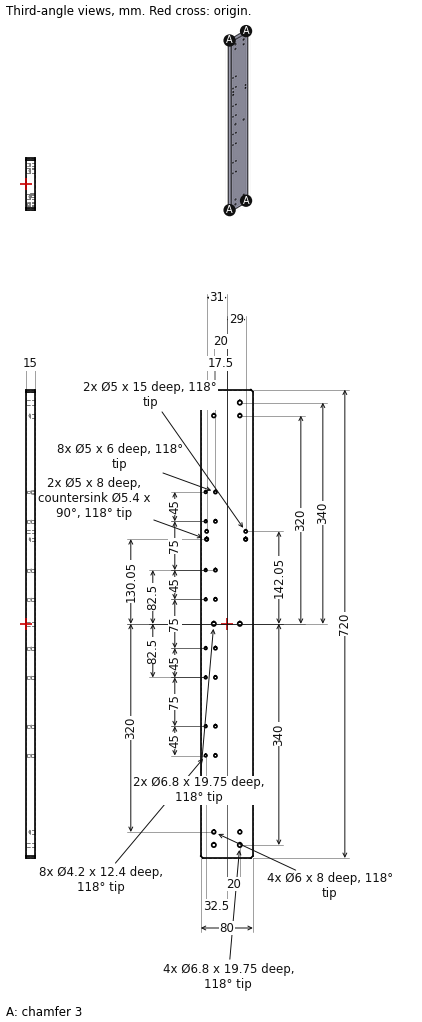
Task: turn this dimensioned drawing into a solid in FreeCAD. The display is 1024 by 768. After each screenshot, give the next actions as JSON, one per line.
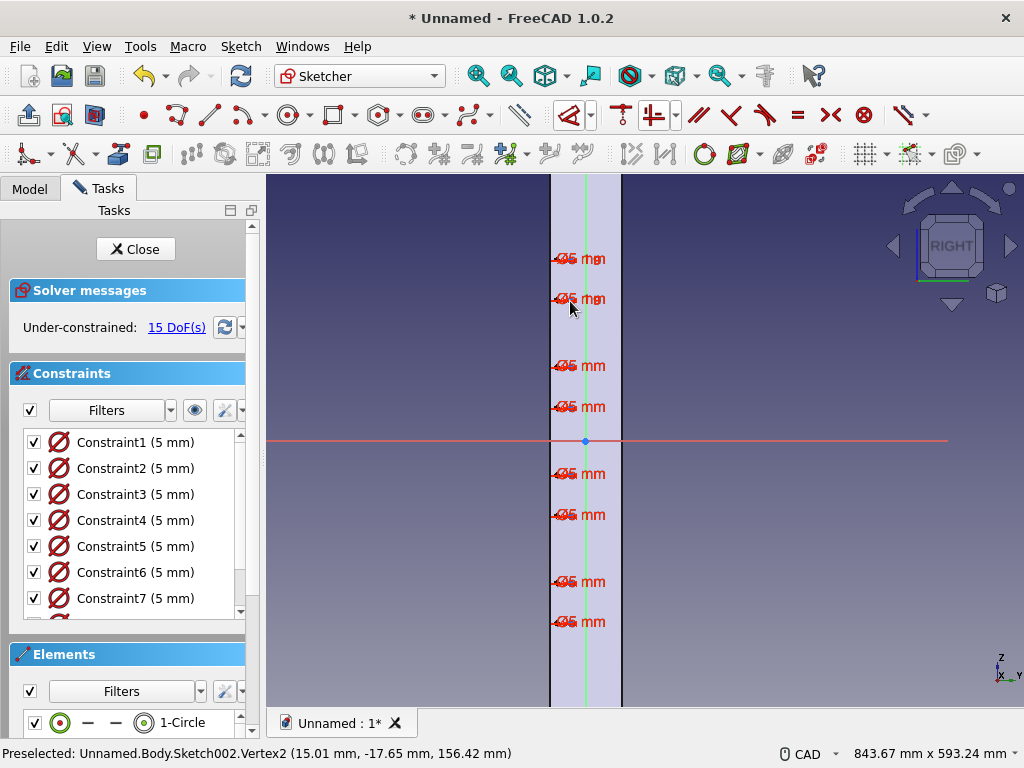
{"action": "left_click", "coordinate": [570, 301]}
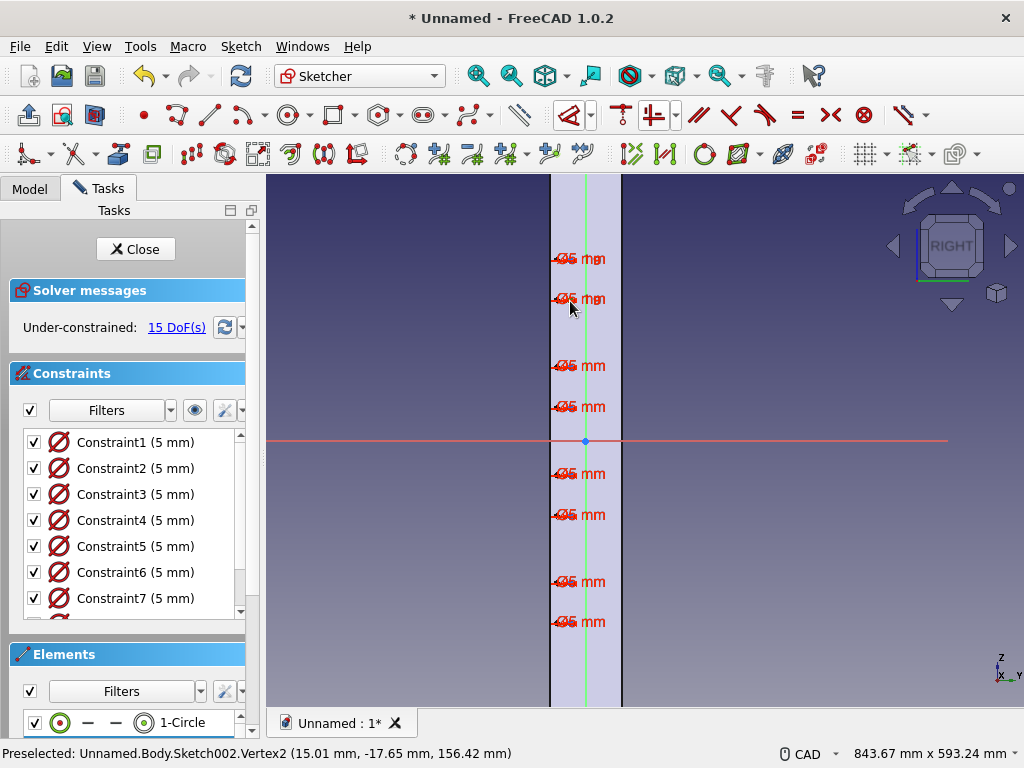
{"action": "left_click", "coordinate": [570, 368]}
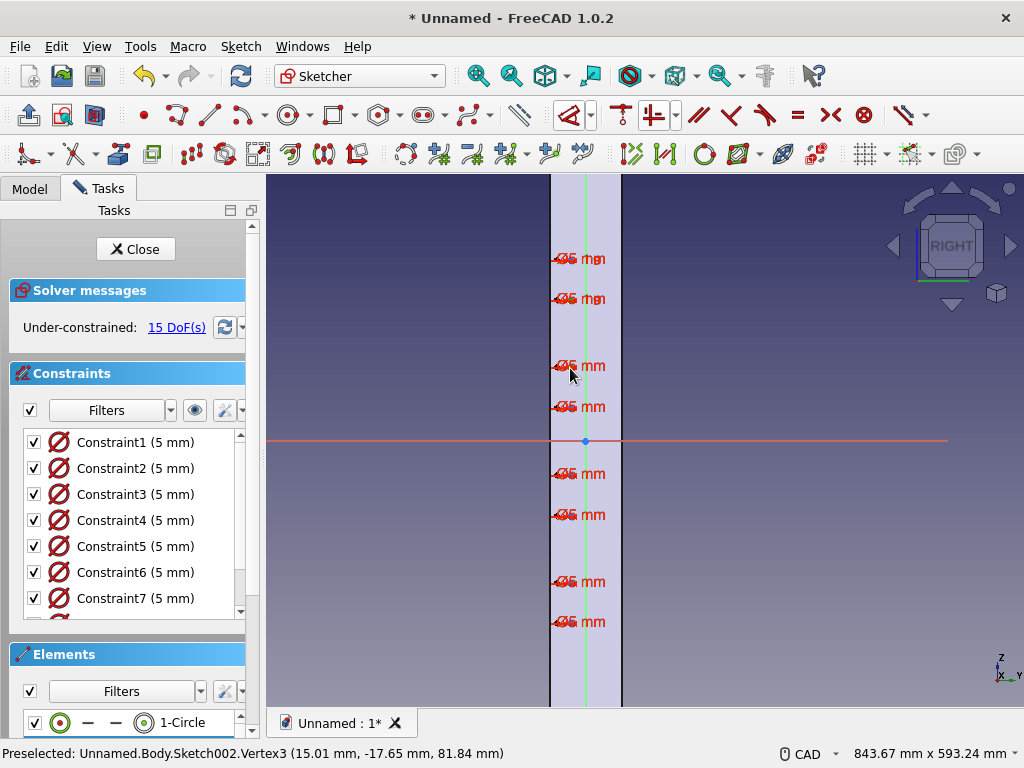
{"action": "key", "text": "v"}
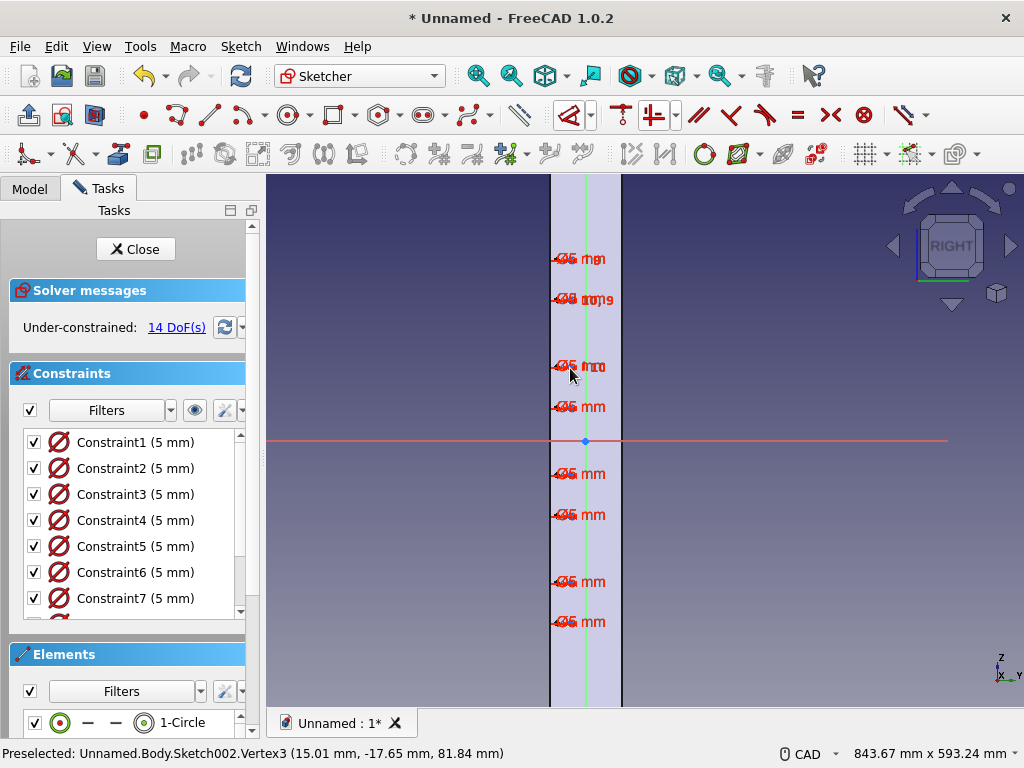
{"action": "left_click", "coordinate": [570, 368]}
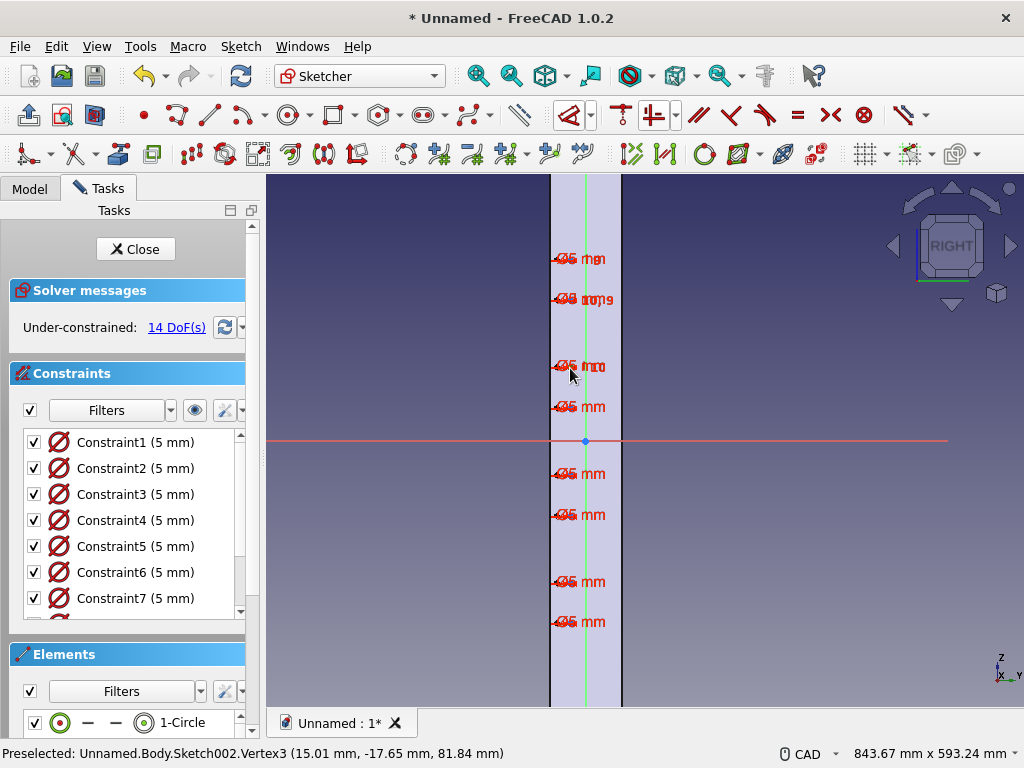
{"action": "left_click", "coordinate": [570, 409]}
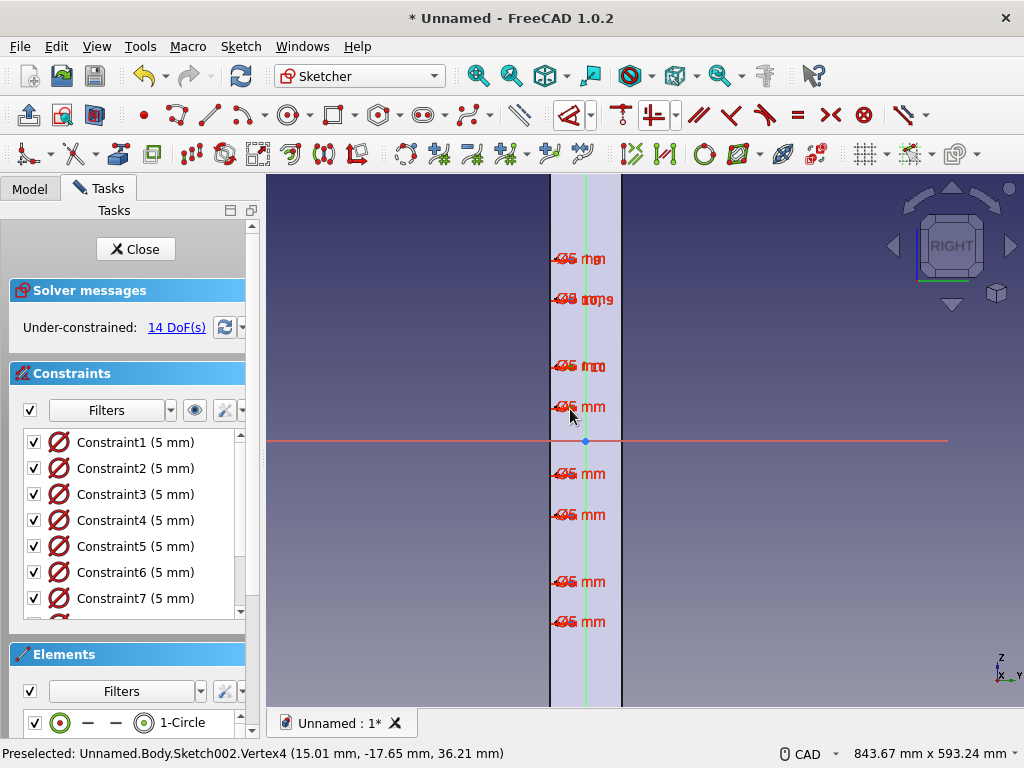
{"action": "left_click", "coordinate": [676, 116]}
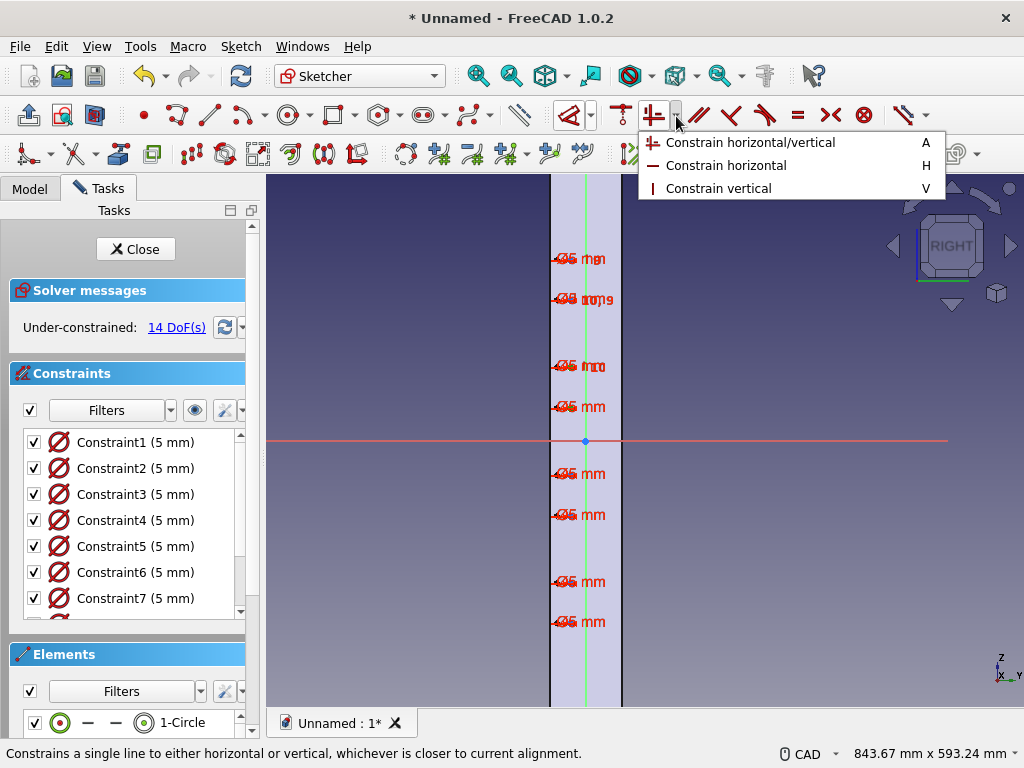
{"action": "left_click", "coordinate": [792, 188]}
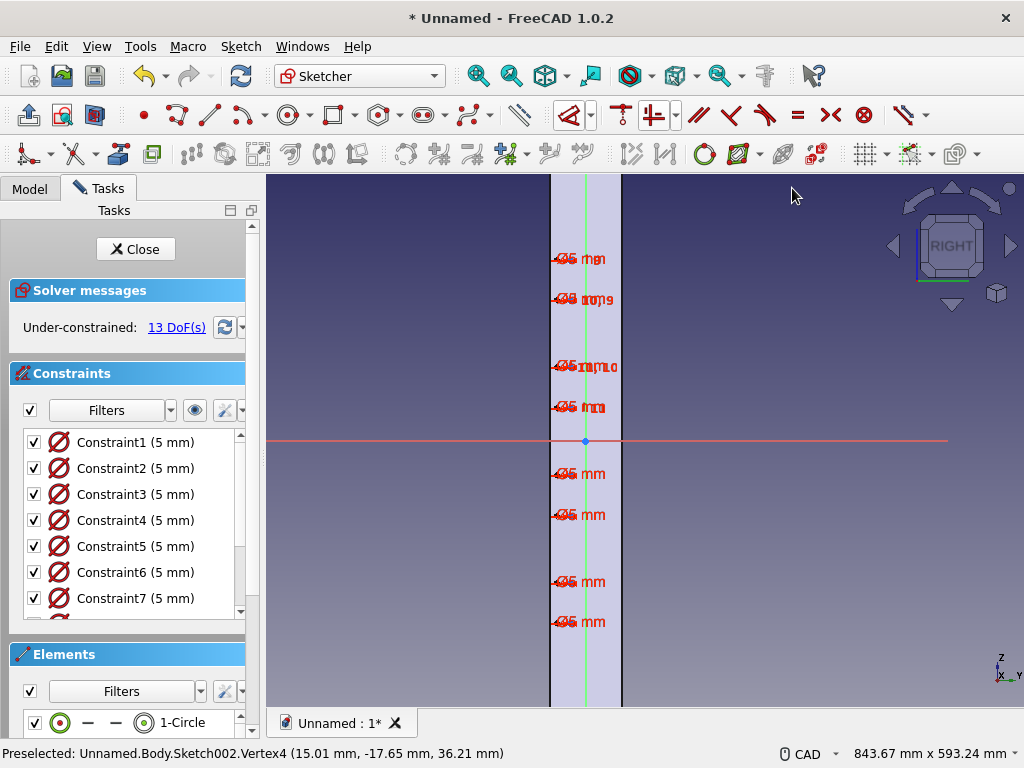
{"action": "left_click", "coordinate": [570, 409]}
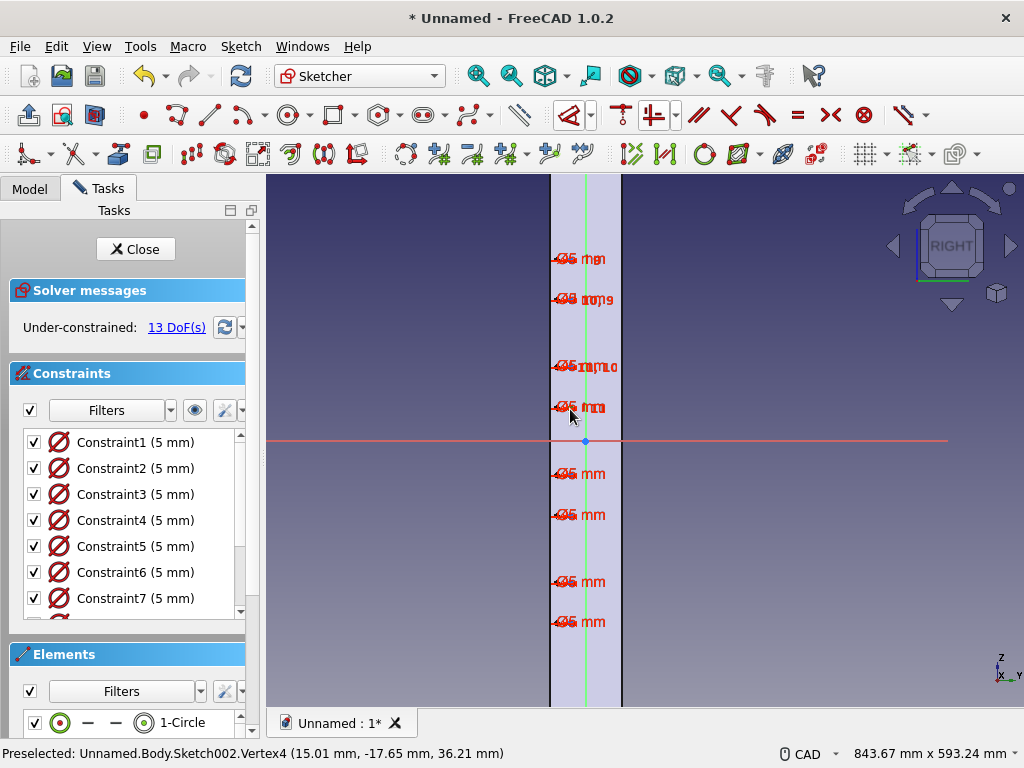
{"action": "left_click", "coordinate": [570, 476]}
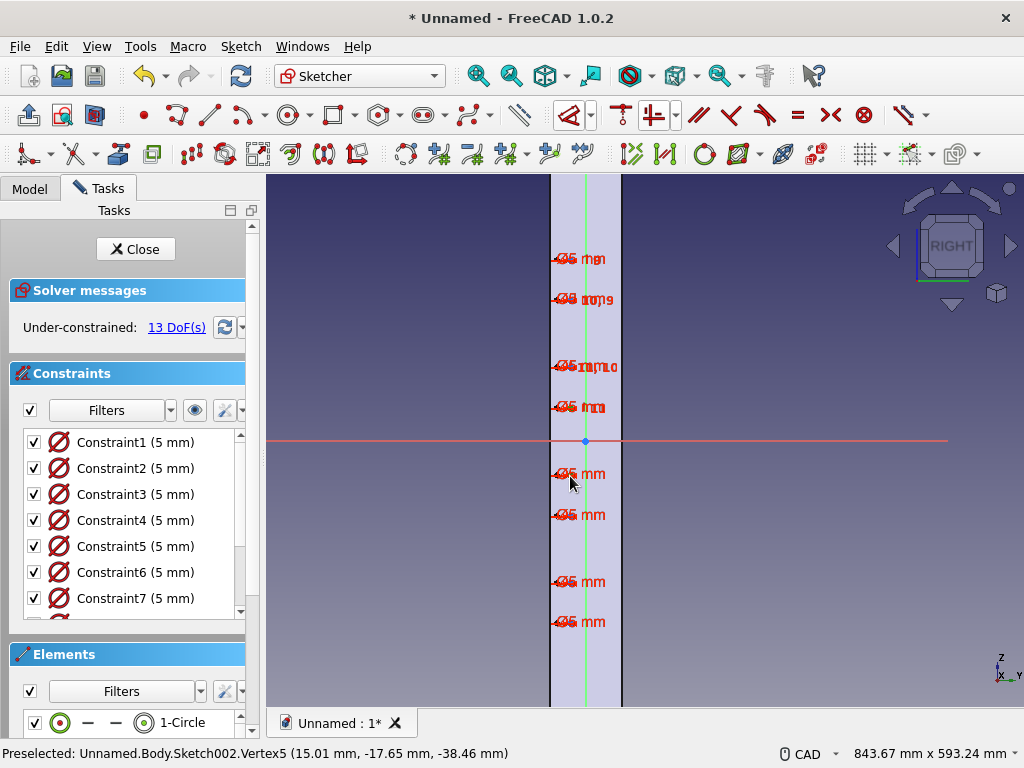
{"action": "left_click", "coordinate": [676, 116]}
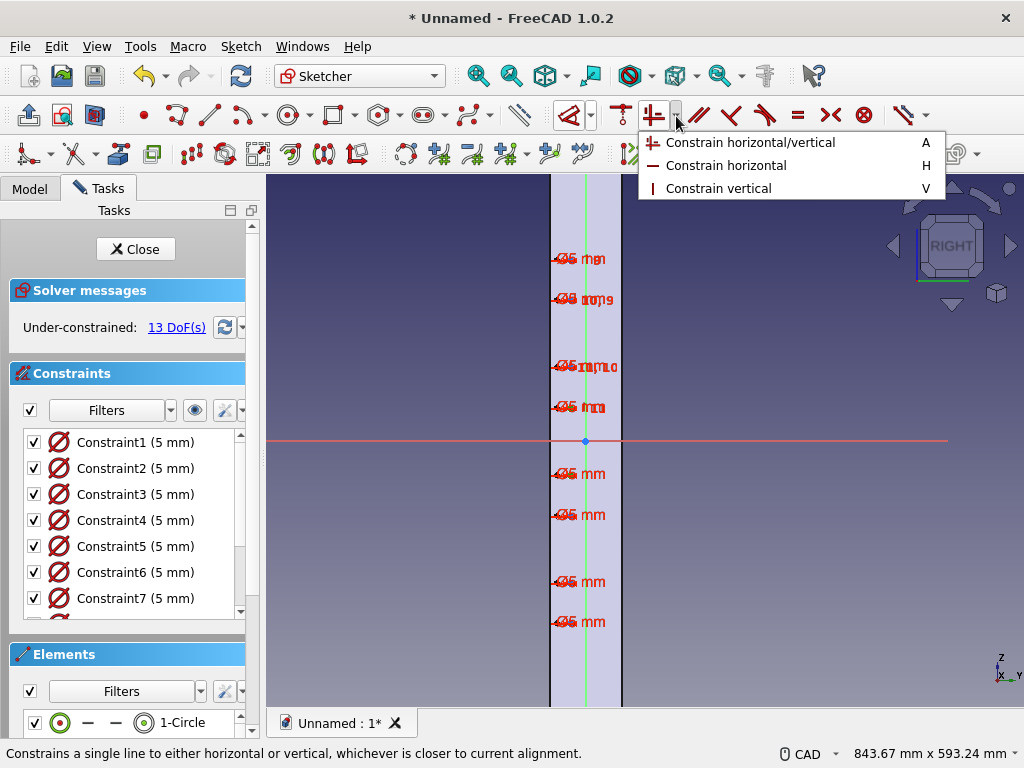
{"action": "left_click", "coordinate": [792, 188]}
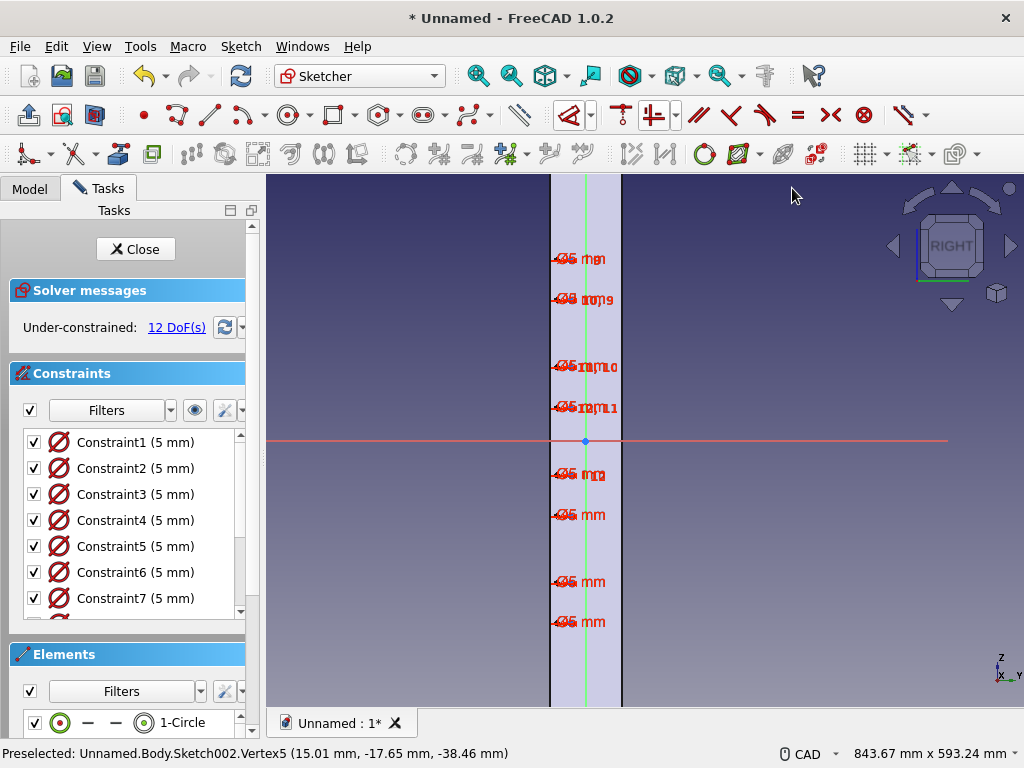
{"action": "left_click", "coordinate": [570, 476]}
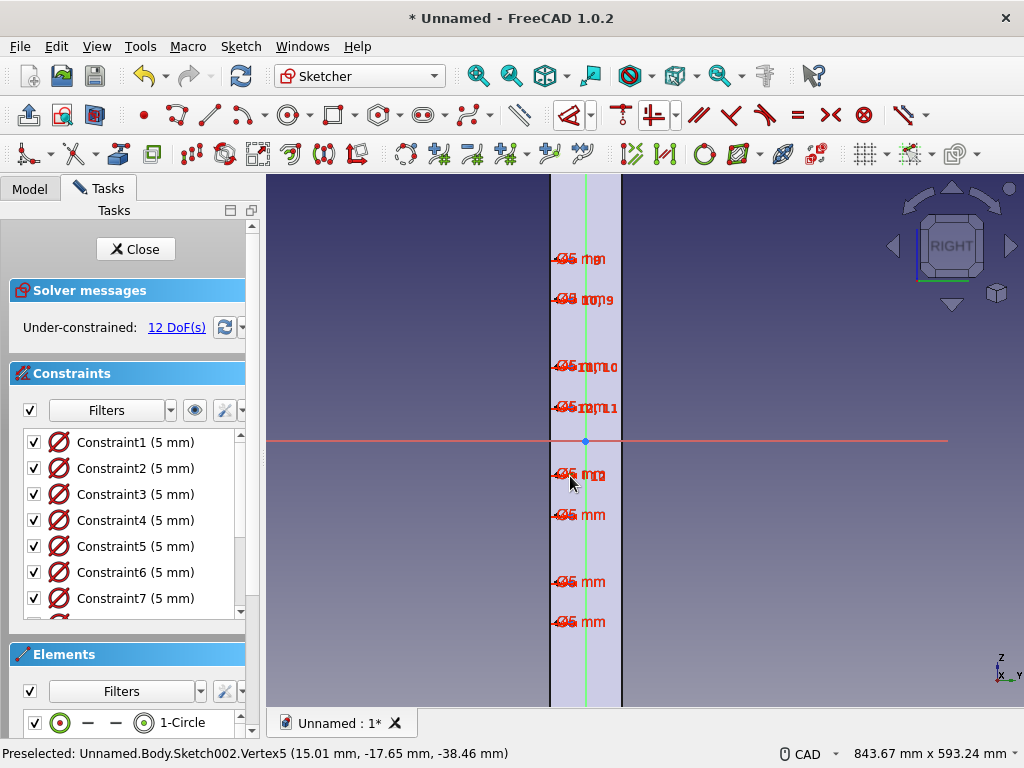
{"action": "left_click", "coordinate": [570, 517]}